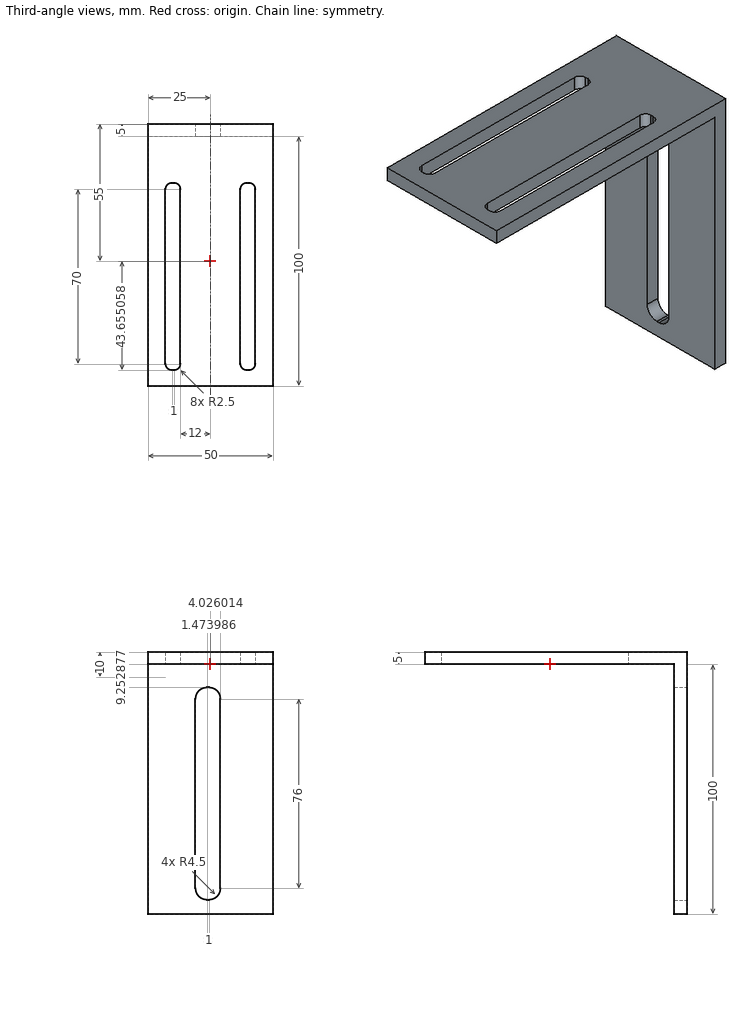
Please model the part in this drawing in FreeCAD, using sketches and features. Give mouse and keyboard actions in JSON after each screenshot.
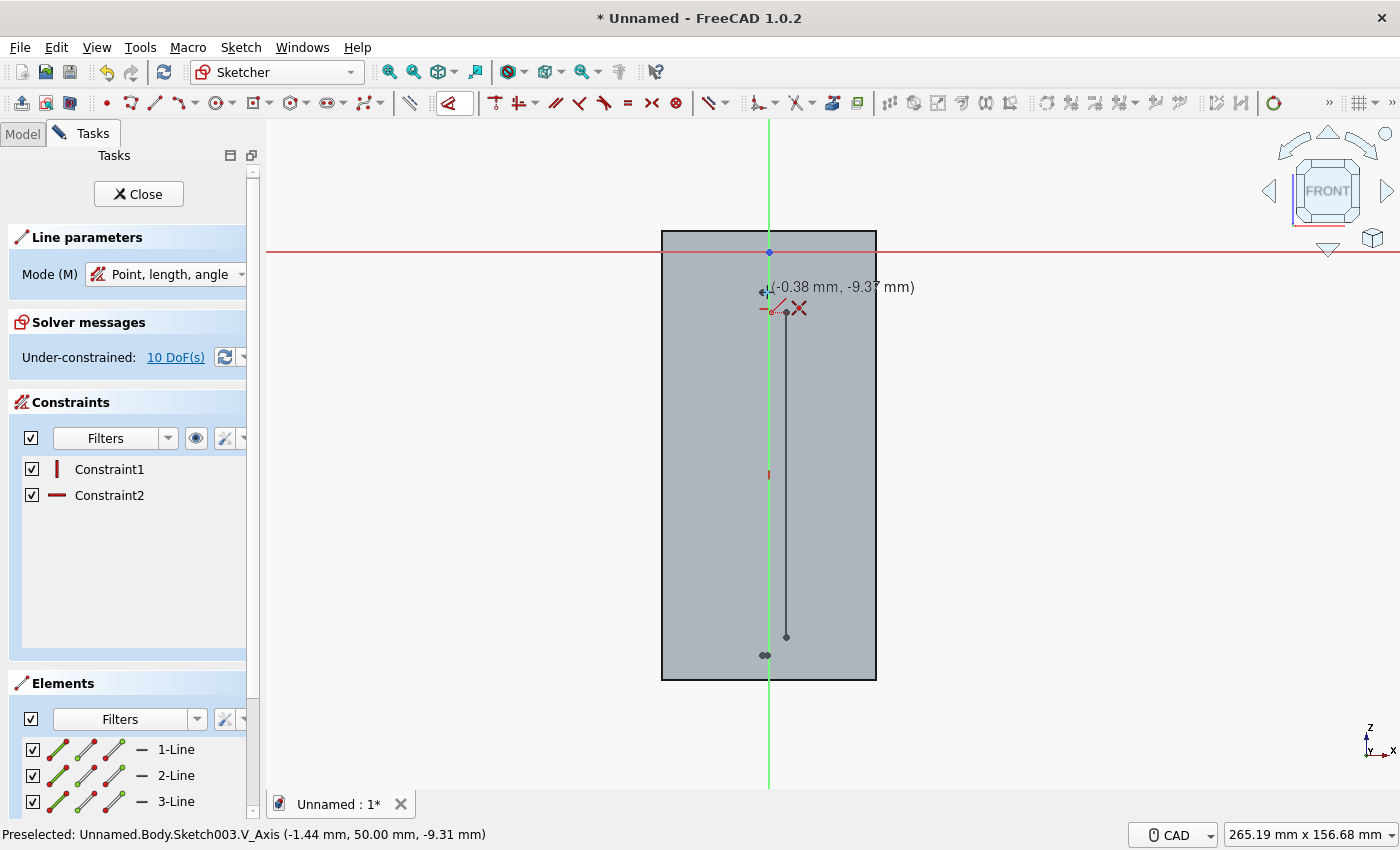
{"action": "left_click", "coordinate": [743, 311]}
{"action": "left_click", "coordinate": [743, 636]}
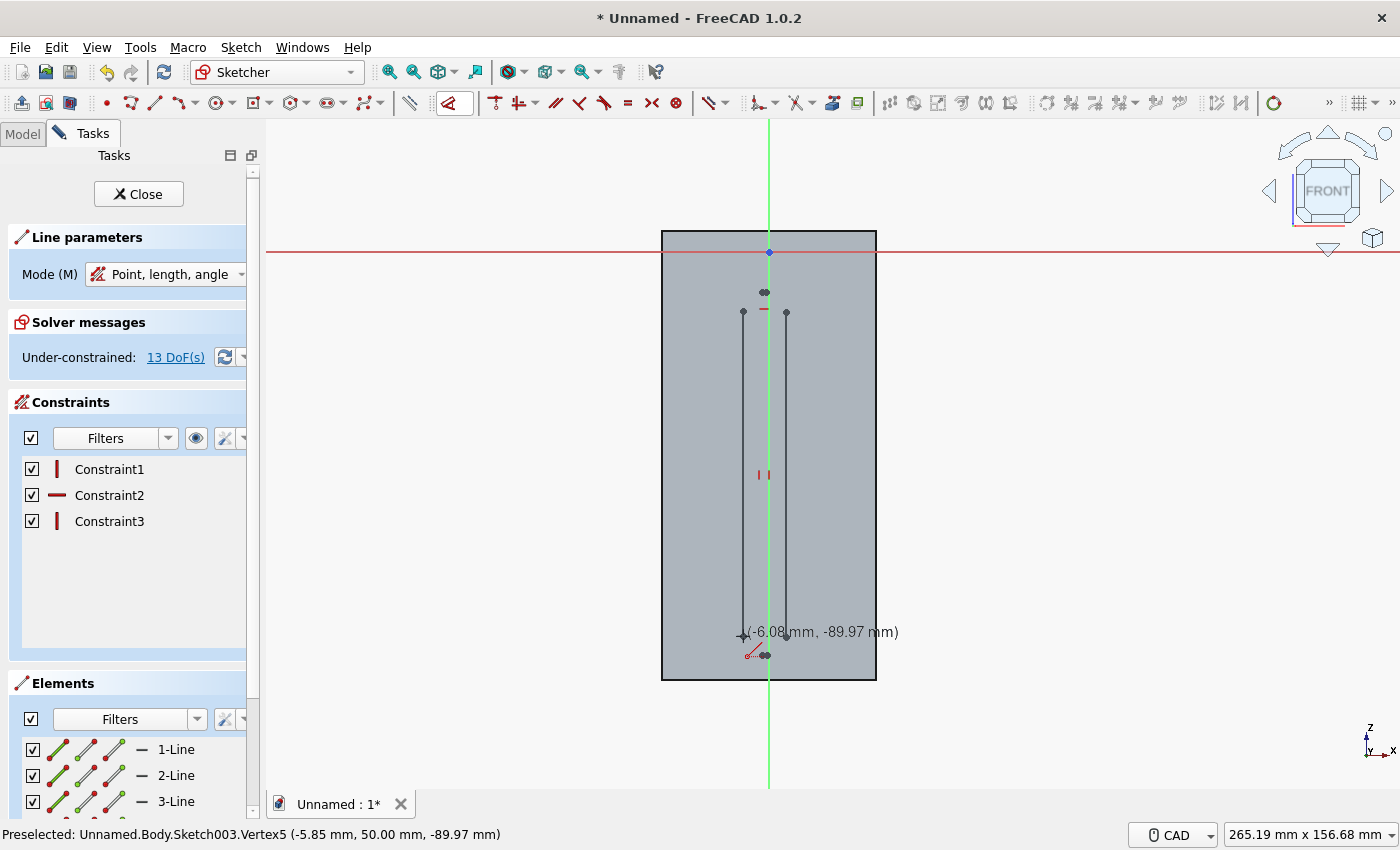
{"action": "key", "text": "g 3 a"}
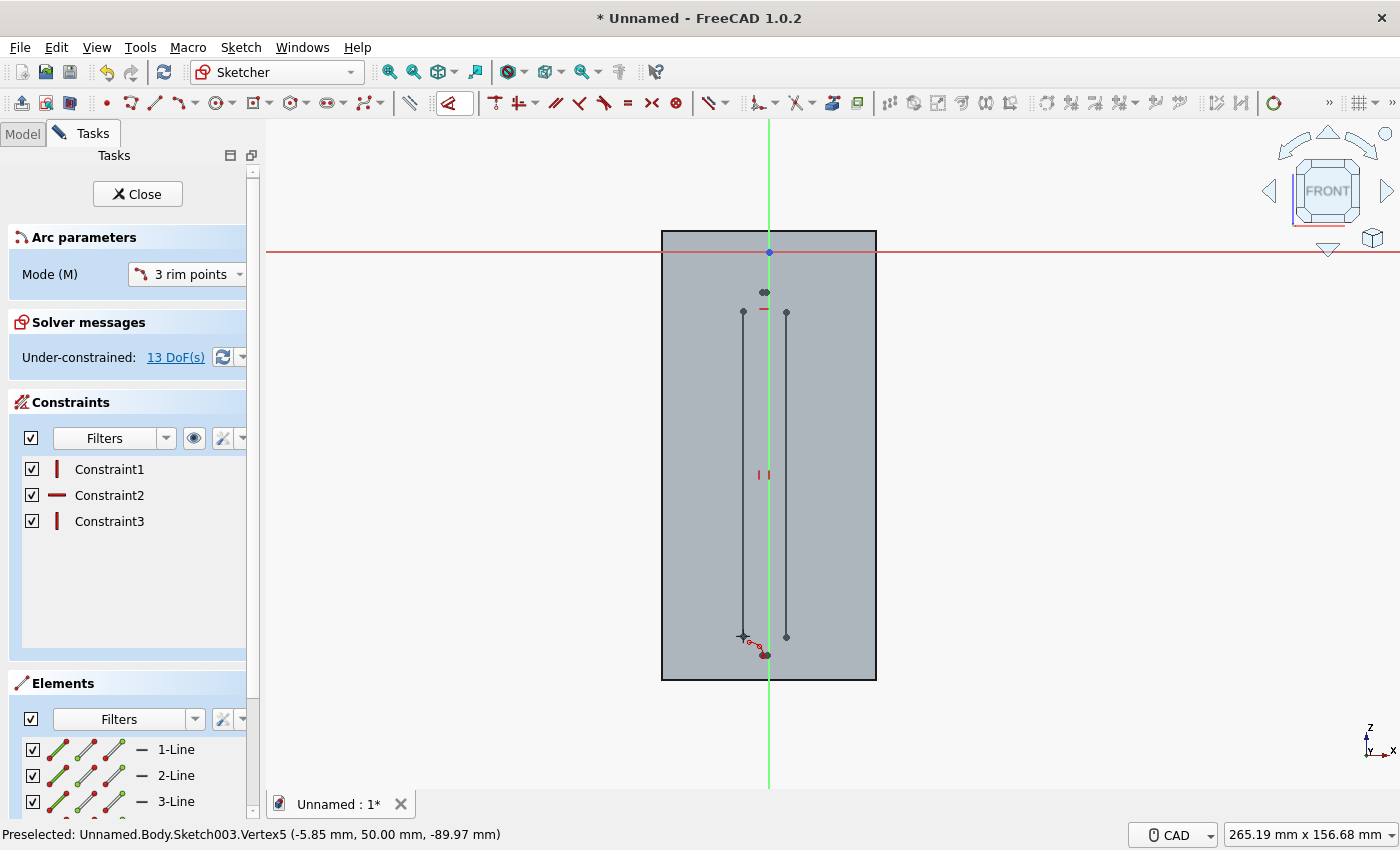
{"action": "scroll", "coordinate": [767, 655], "scroll_direction": "up", "scroll_amount": 11}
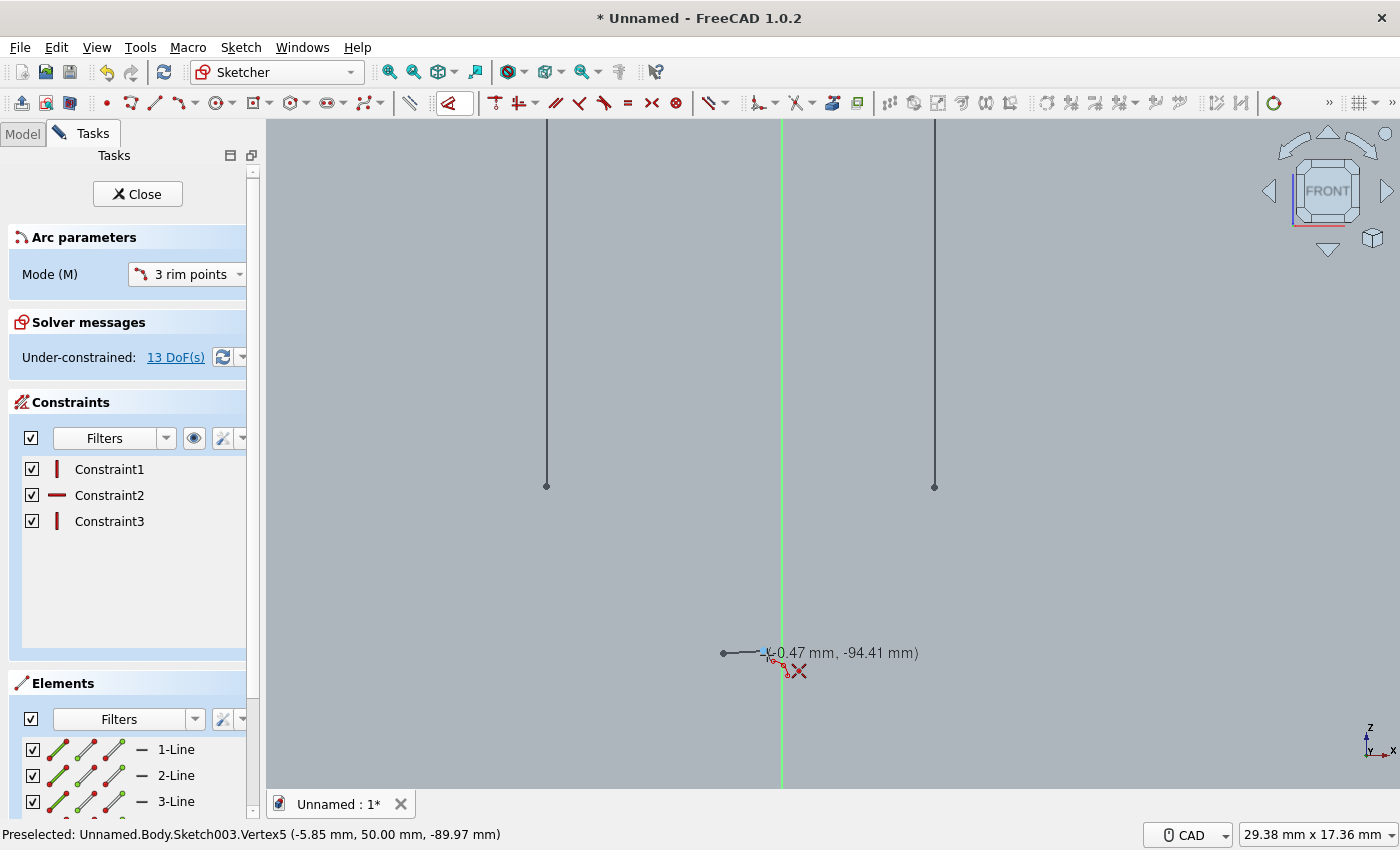
{"action": "left_click", "coordinate": [764, 651]}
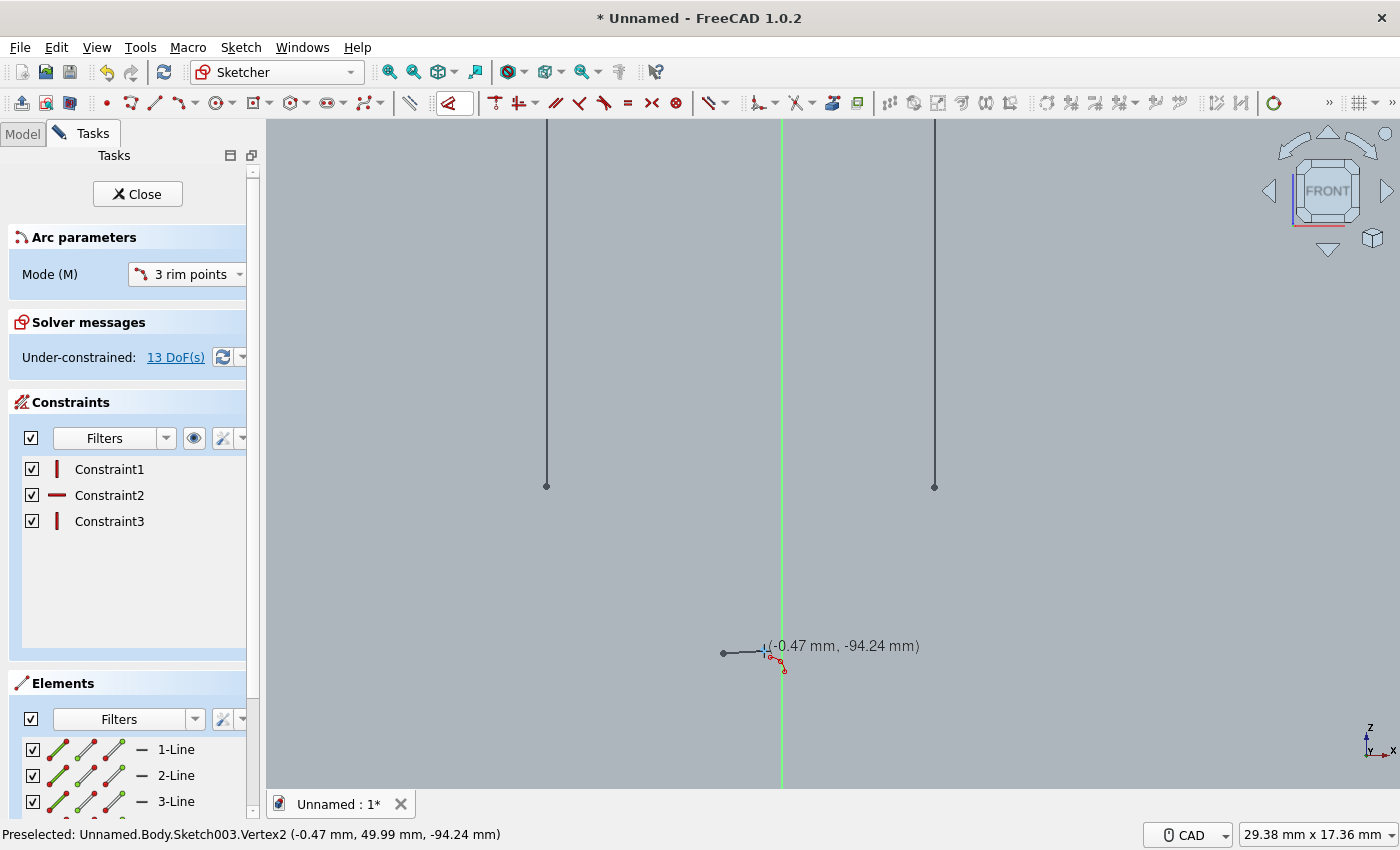
{"action": "scroll", "coordinate": [767, 656], "scroll_direction": "down", "scroll_amount": 11}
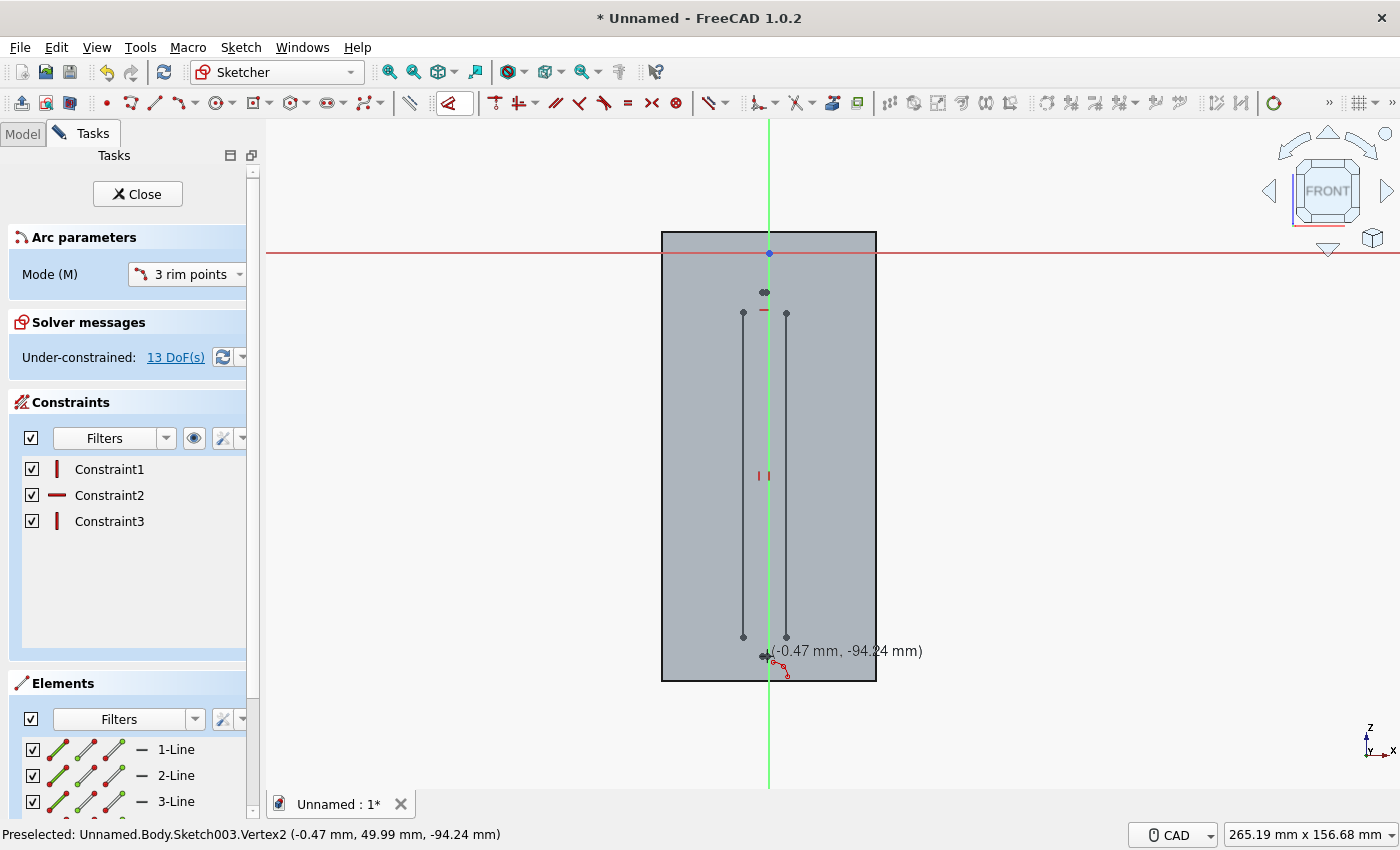
{"action": "left_click", "coordinate": [786, 638]}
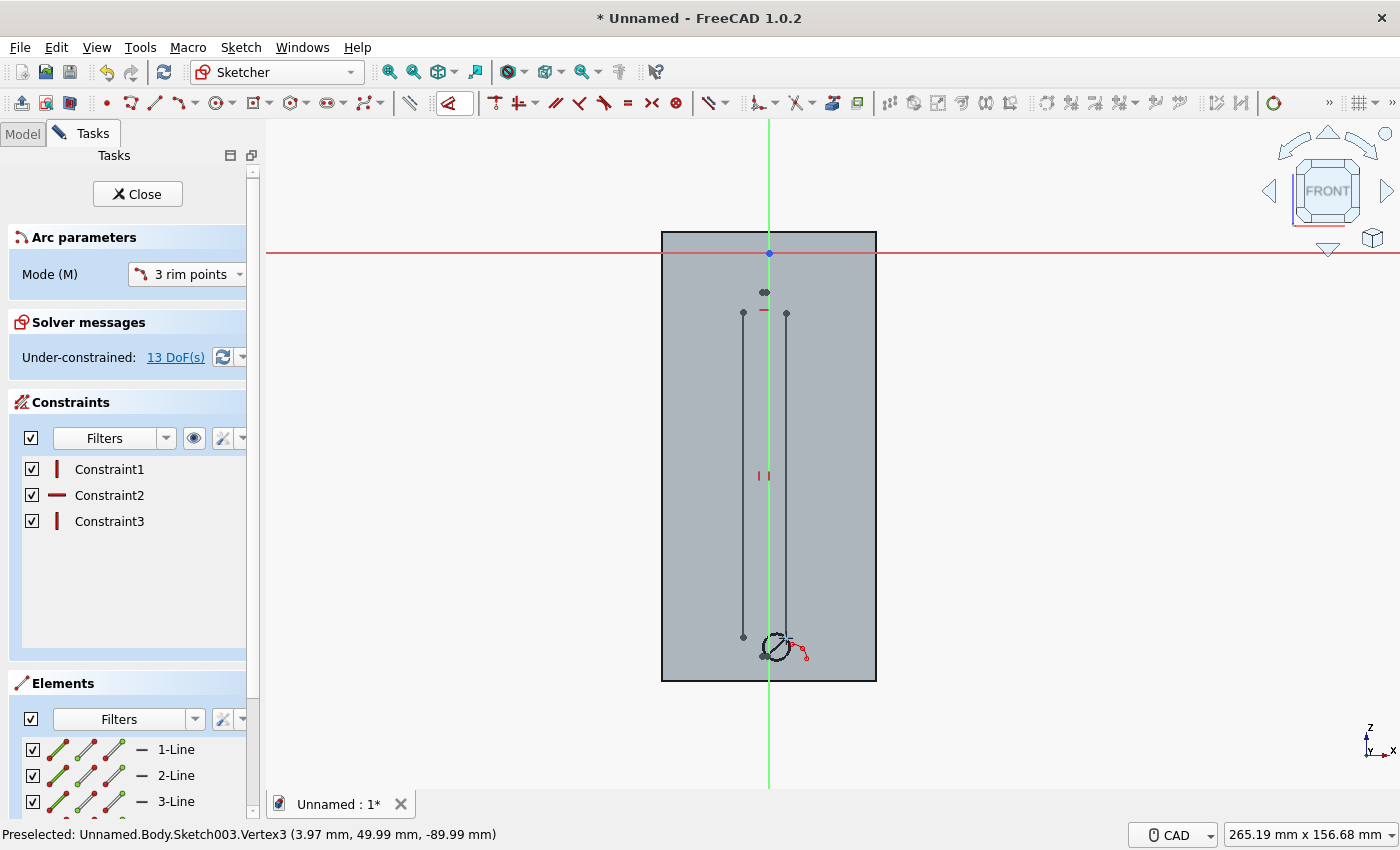
{"action": "scroll", "coordinate": [781, 651], "scroll_direction": "up", "scroll_amount": 6}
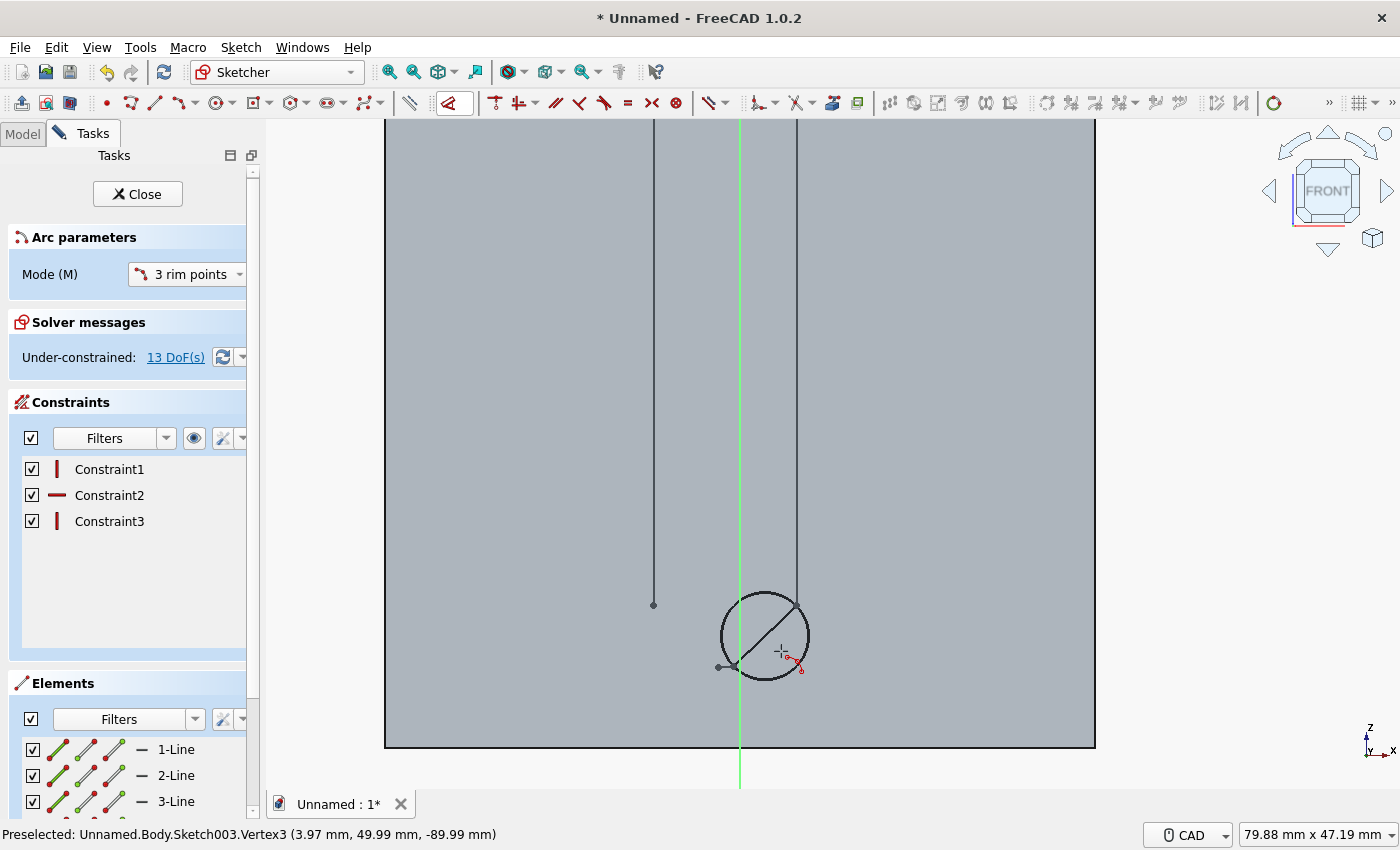
{"action": "left_click", "coordinate": [779, 648]}